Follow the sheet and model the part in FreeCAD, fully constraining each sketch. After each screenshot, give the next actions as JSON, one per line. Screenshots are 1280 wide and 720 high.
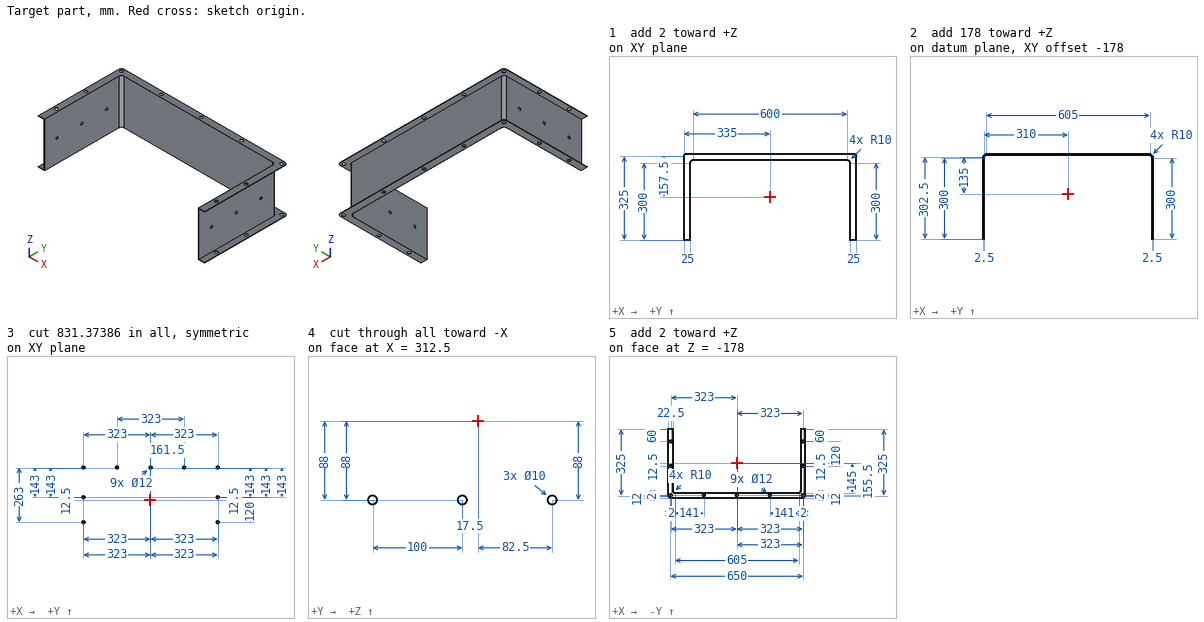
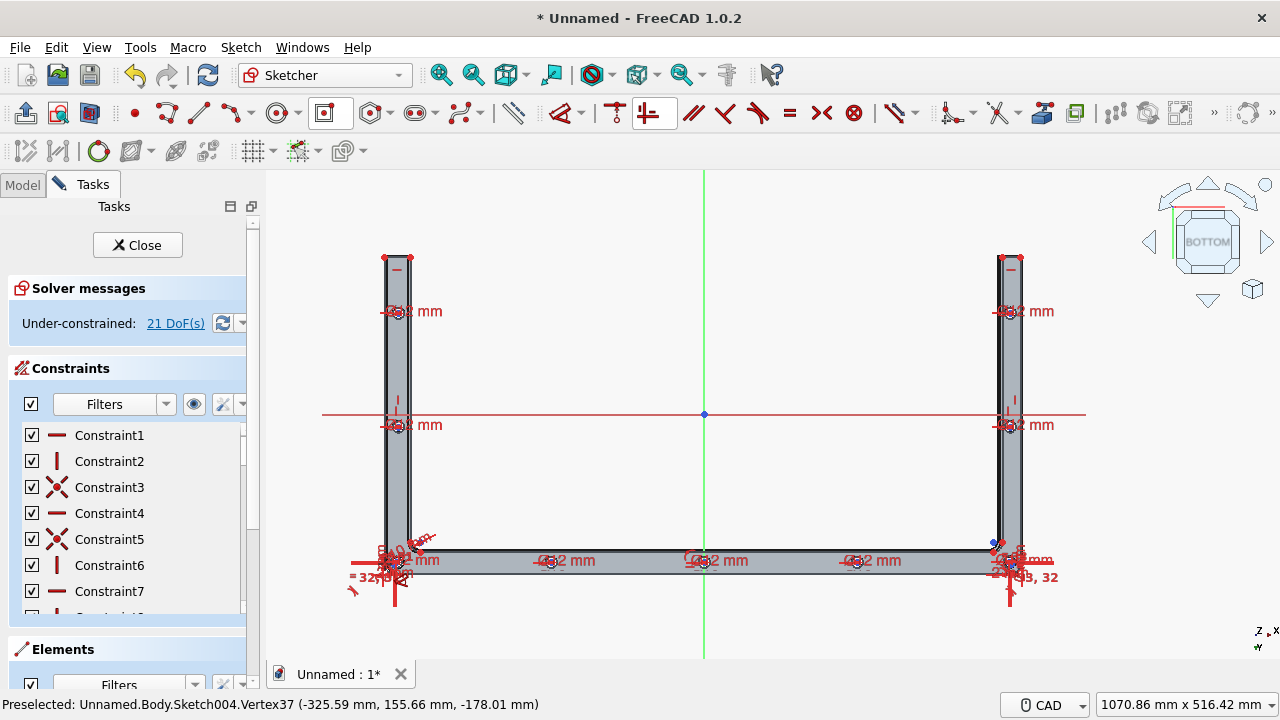
{"action": "left_click", "coordinate": [821, 552]}
{"action": "left_click", "coordinate": [575, 518]}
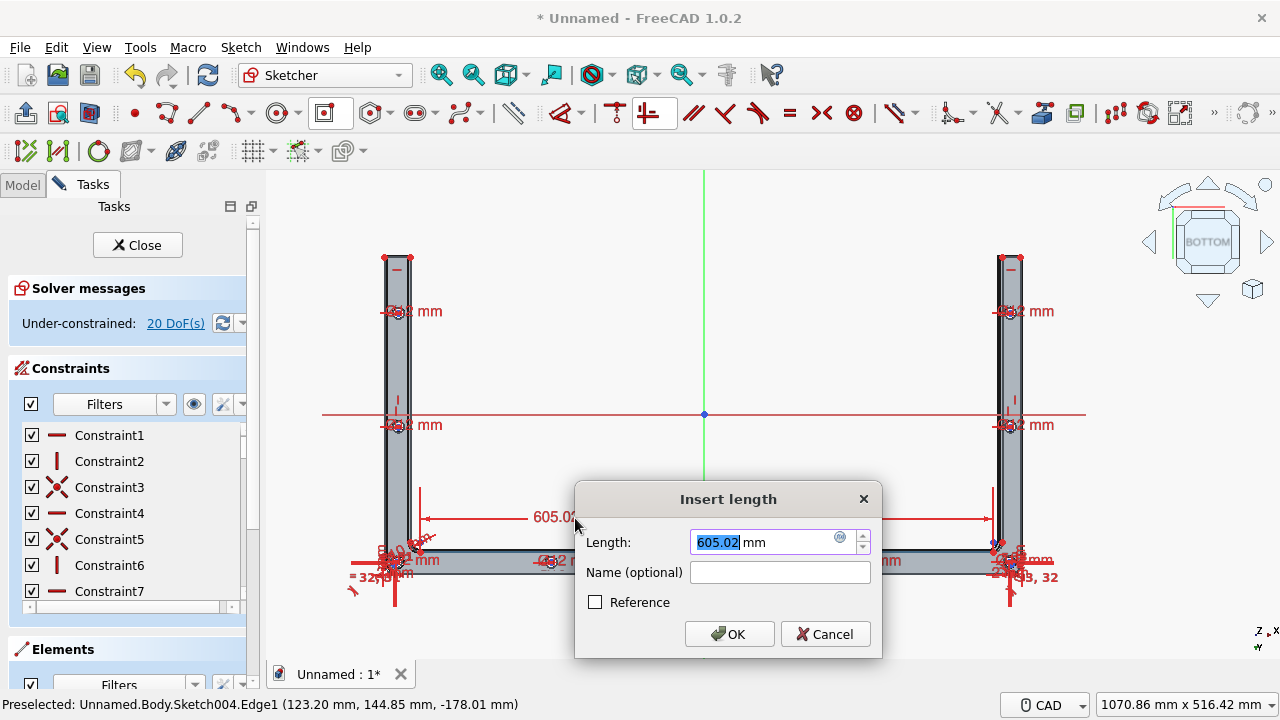
{"action": "type", "text": "605"}
{"action": "key", "text": "Return"}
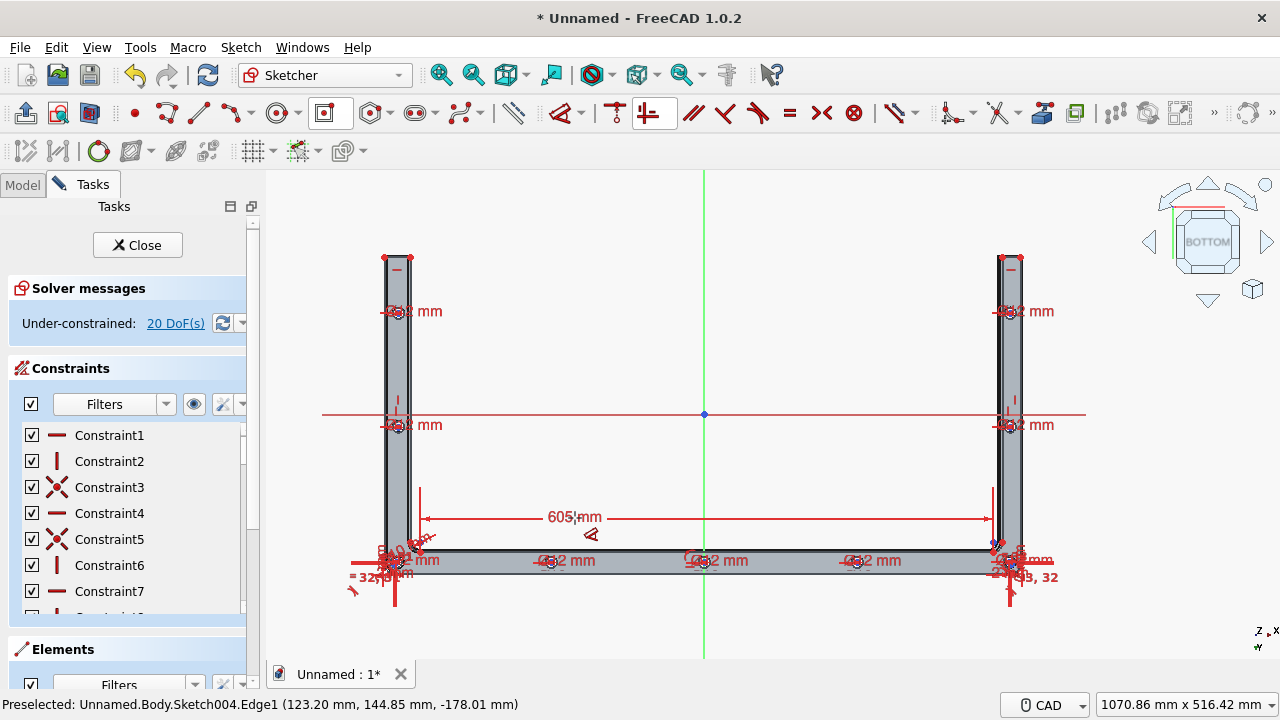
{"action": "left_click", "coordinate": [385, 349]}
{"action": "left_click", "coordinate": [351, 340]}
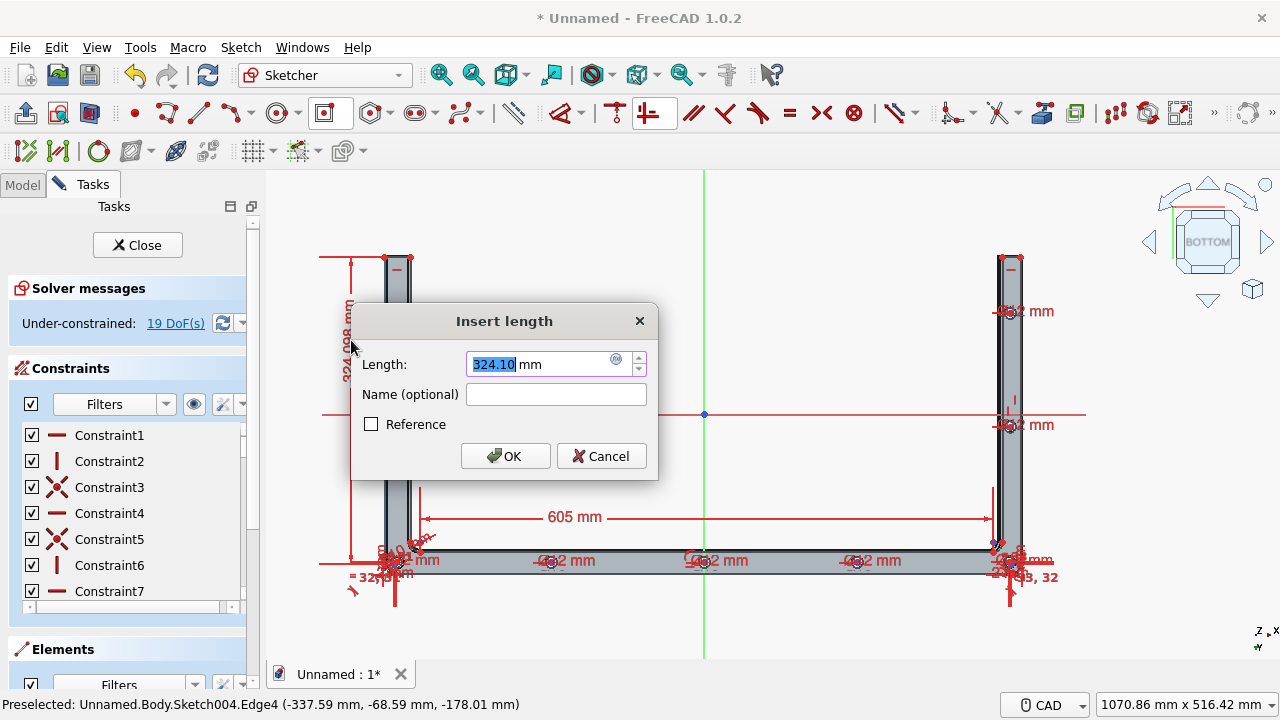
{"action": "type", "text": "325"}
{"action": "key", "text": "Return"}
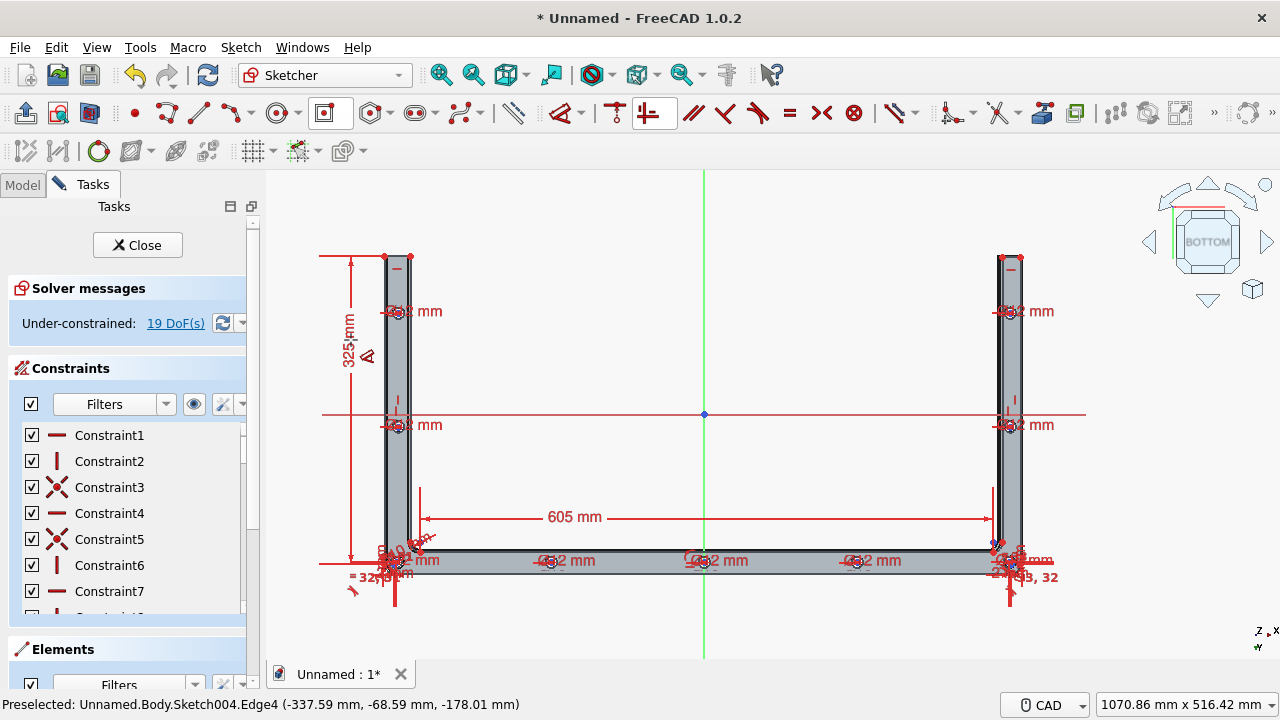
{"action": "left_click", "coordinate": [579, 574]}
{"action": "left_click", "coordinate": [561, 608]}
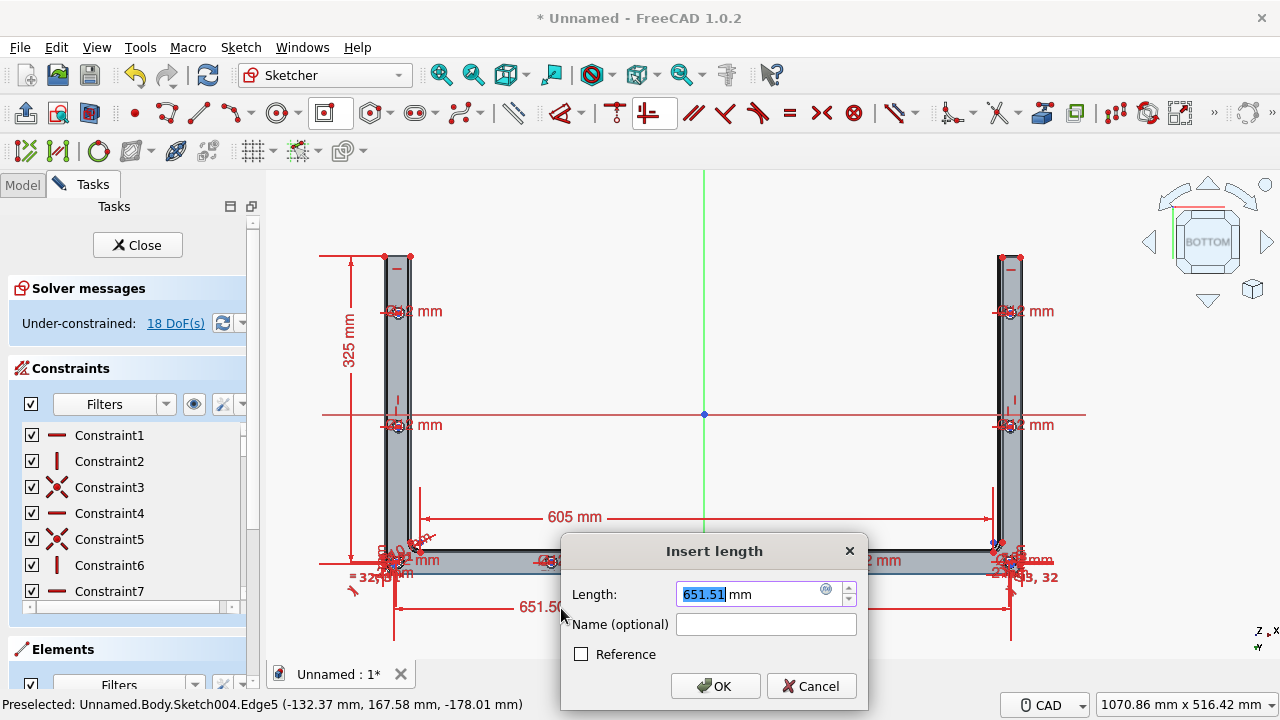
{"action": "type", "text": "650"}
{"action": "key", "text": "Return"}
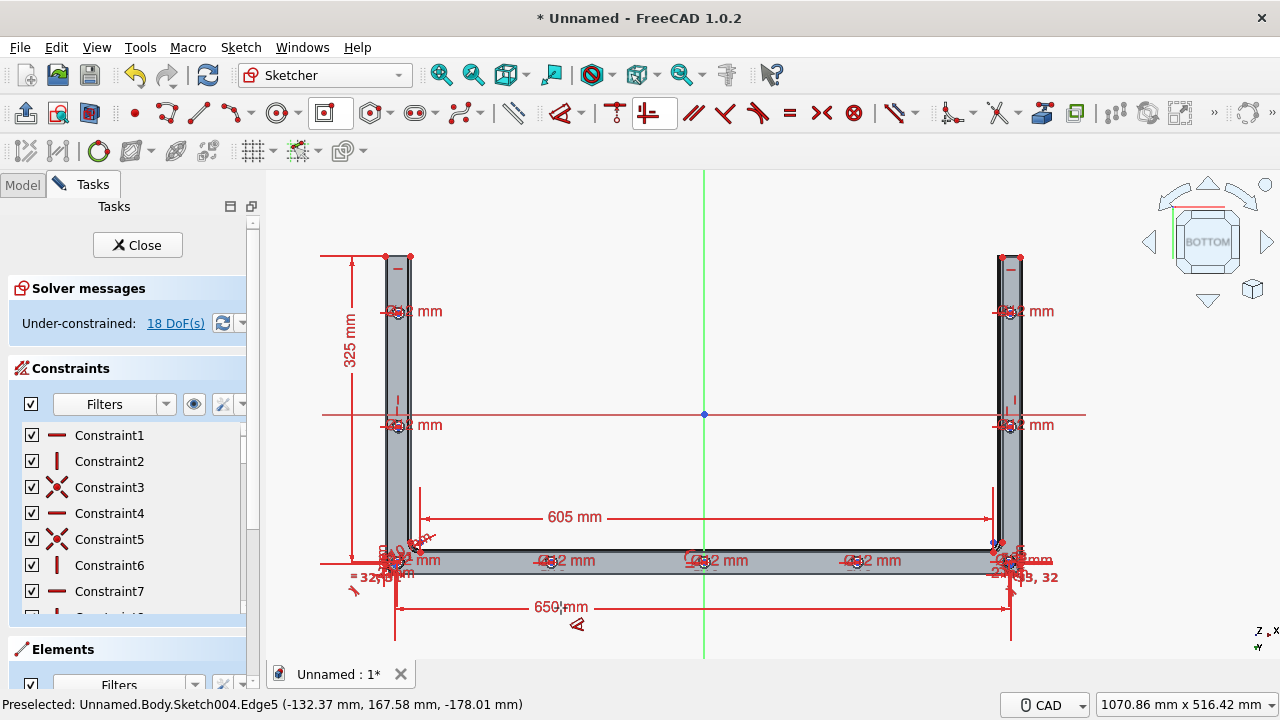
{"action": "left_click", "coordinate": [1020, 472]}
{"action": "left_click", "coordinate": [1054, 340]}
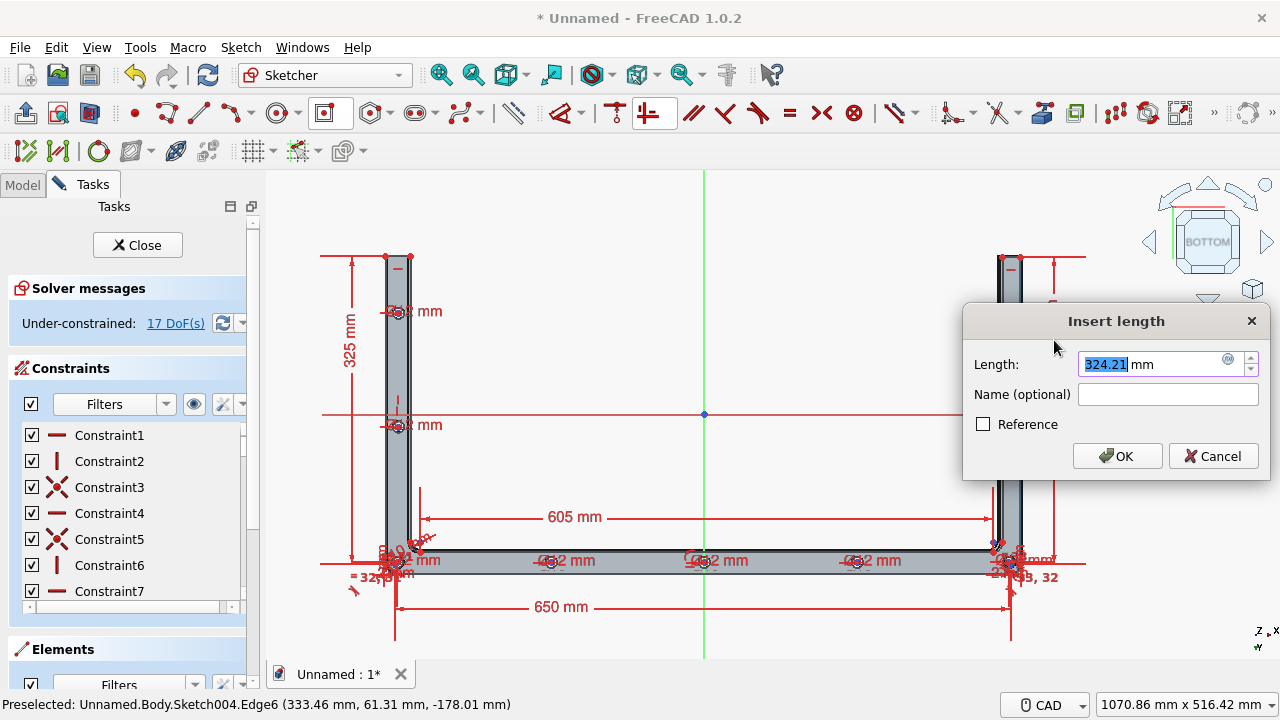
{"action": "type", "text": "325"}
{"action": "key", "text": "Return"}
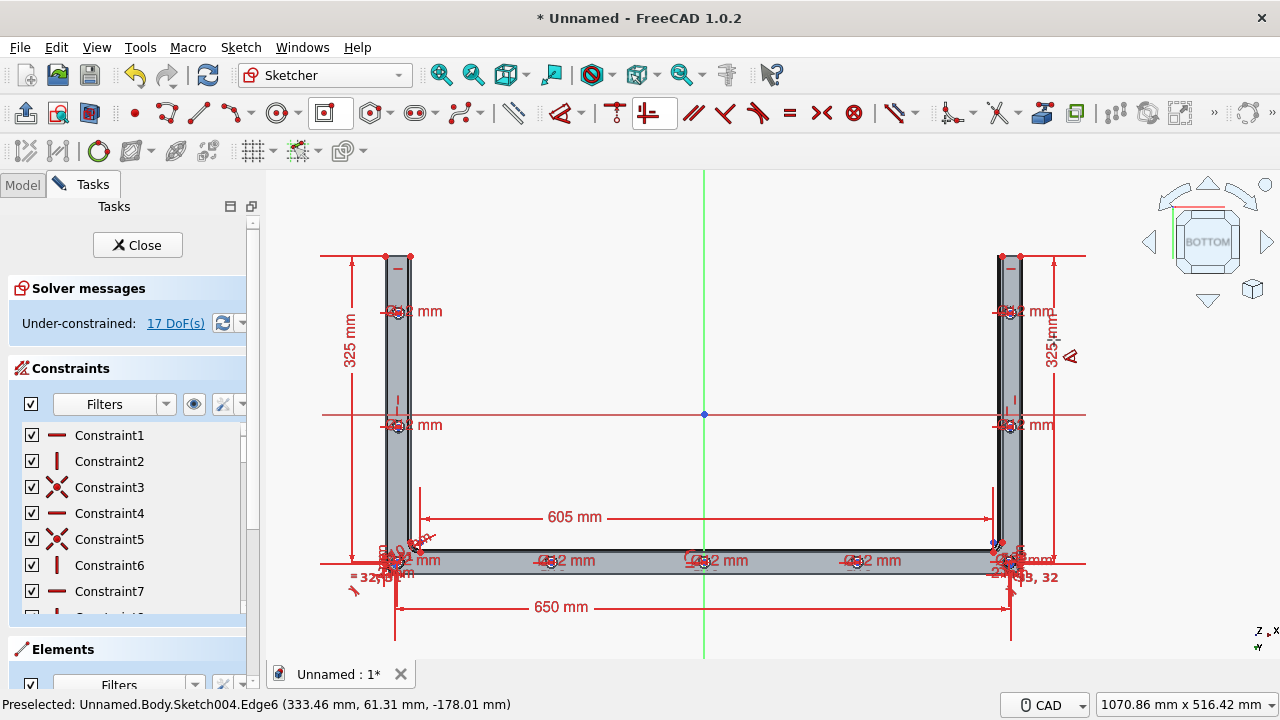
{"action": "left_click", "coordinate": [1010, 313]}
{"action": "left_click", "coordinate": [857, 279]}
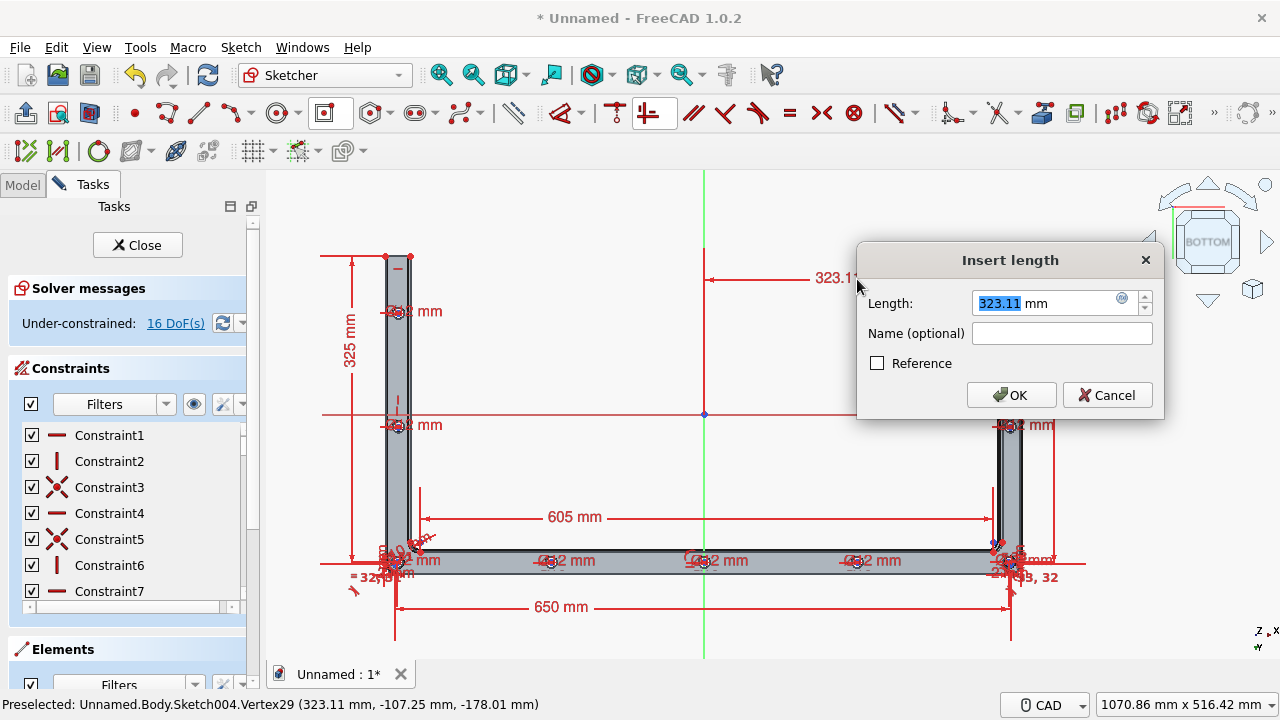
{"action": "type", "text": "323"}
{"action": "key", "text": "Return"}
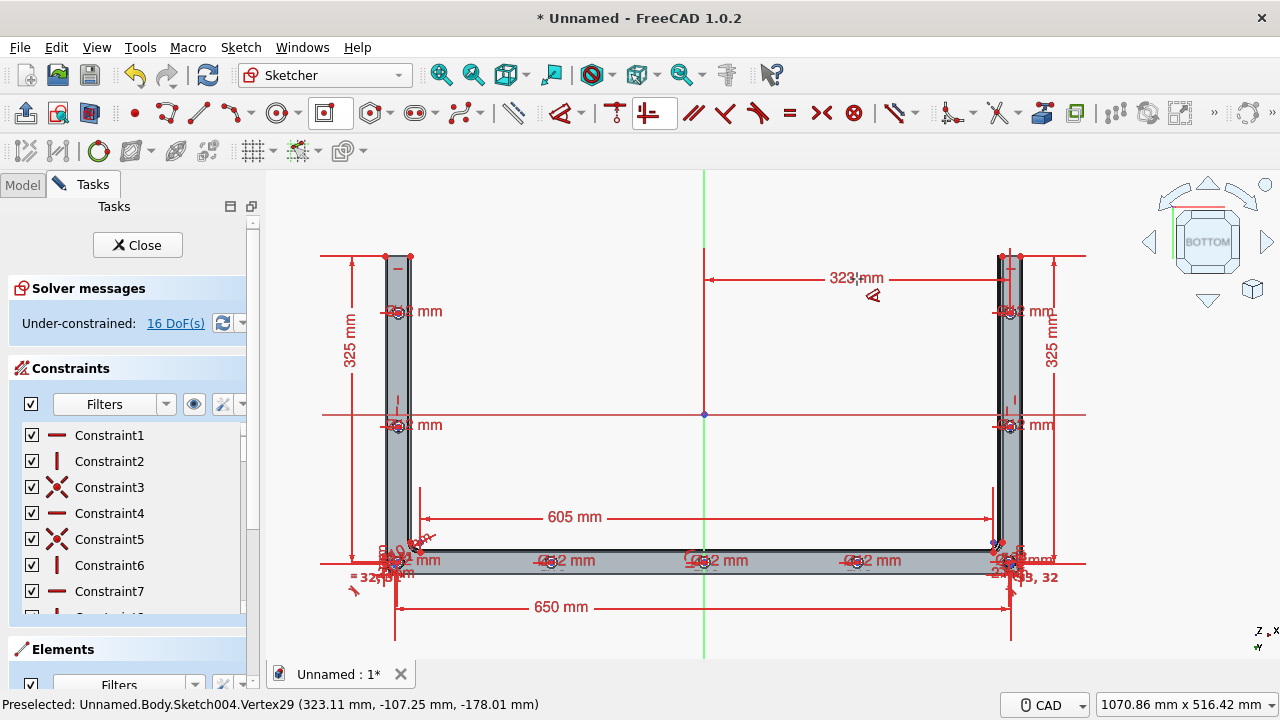
{"action": "left_click", "coordinate": [1010, 427]}
{"action": "left_click", "coordinate": [857, 461]}